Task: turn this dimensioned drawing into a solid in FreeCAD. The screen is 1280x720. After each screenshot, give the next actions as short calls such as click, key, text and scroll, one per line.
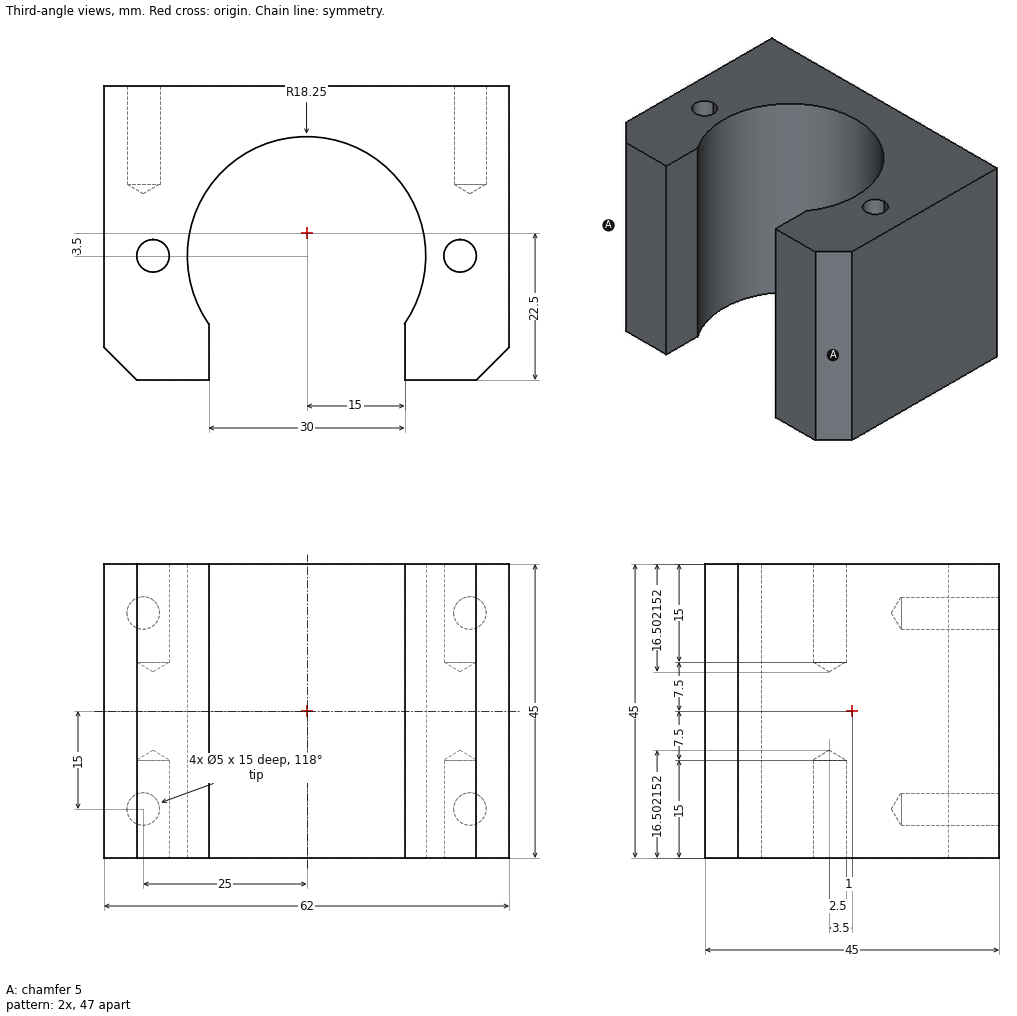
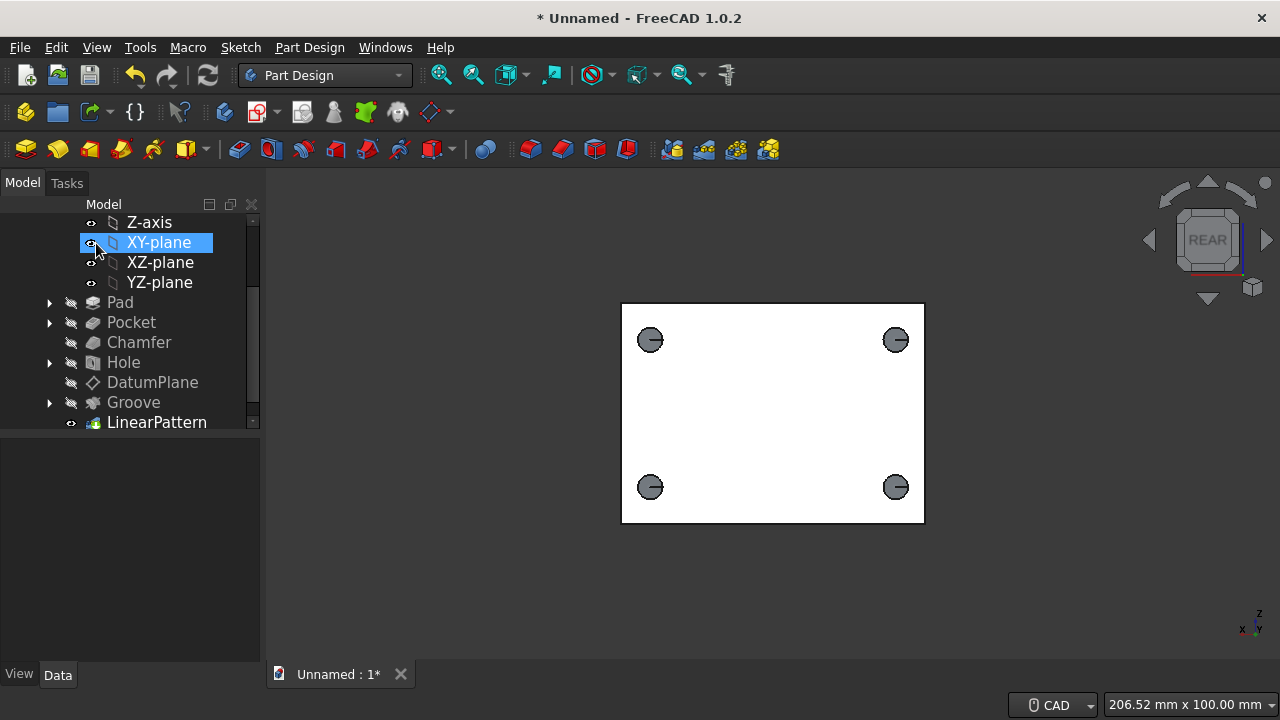
click(116, 403)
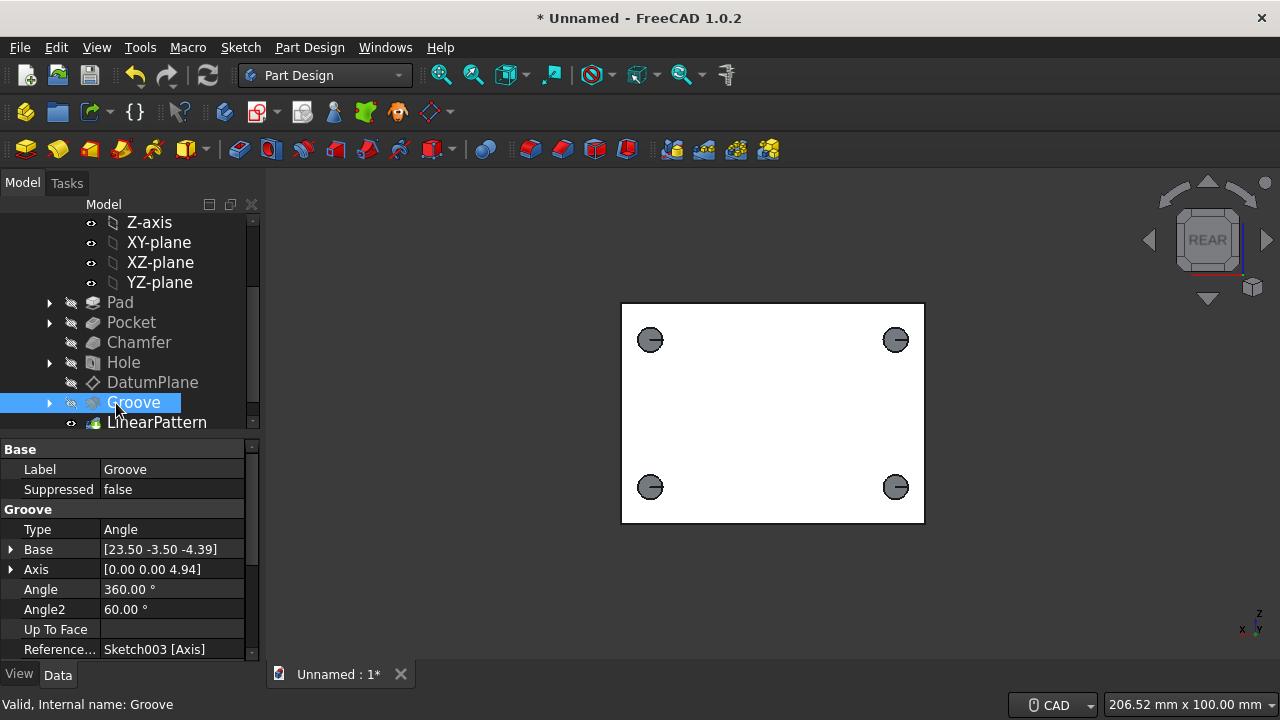
click(672, 150)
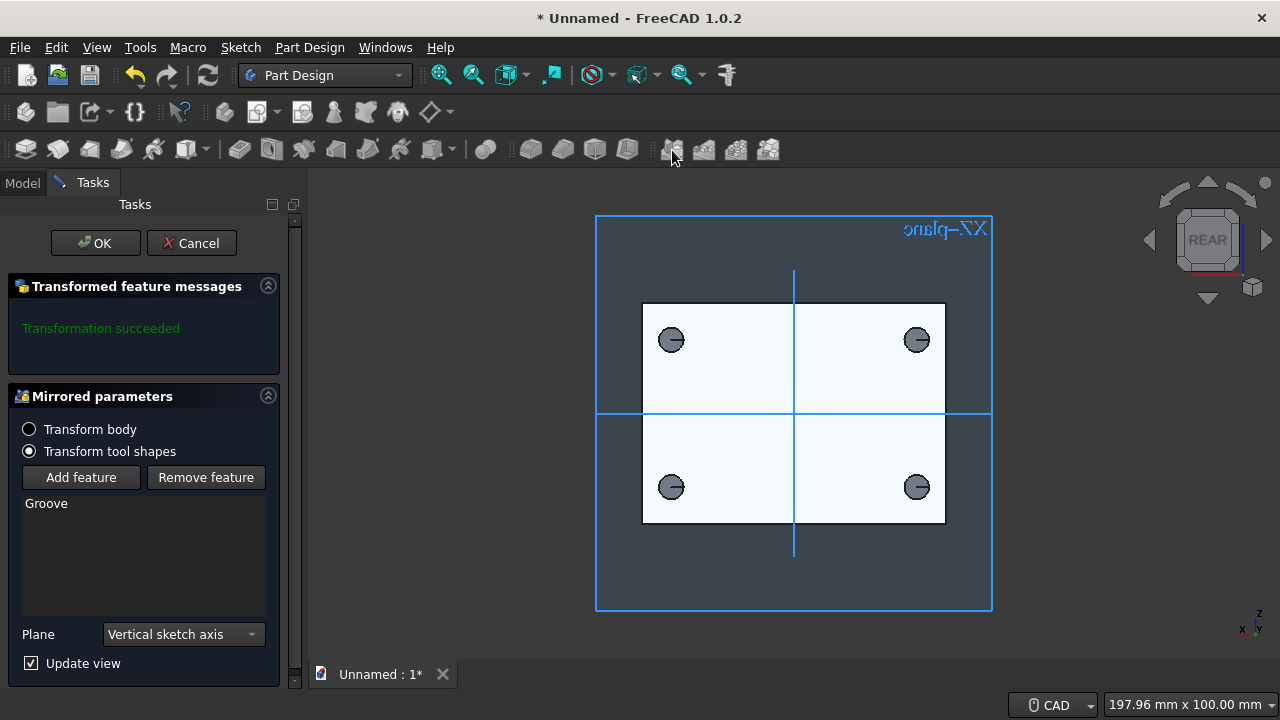
click(184, 634)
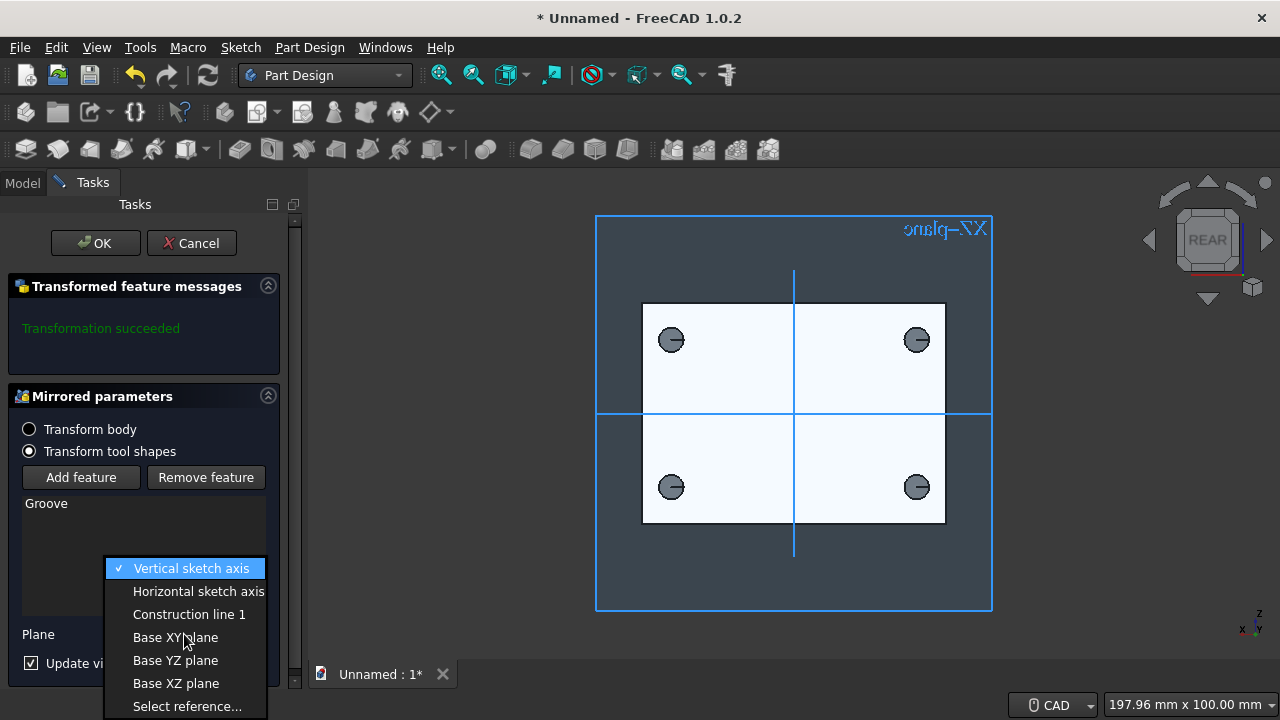
click(184, 638)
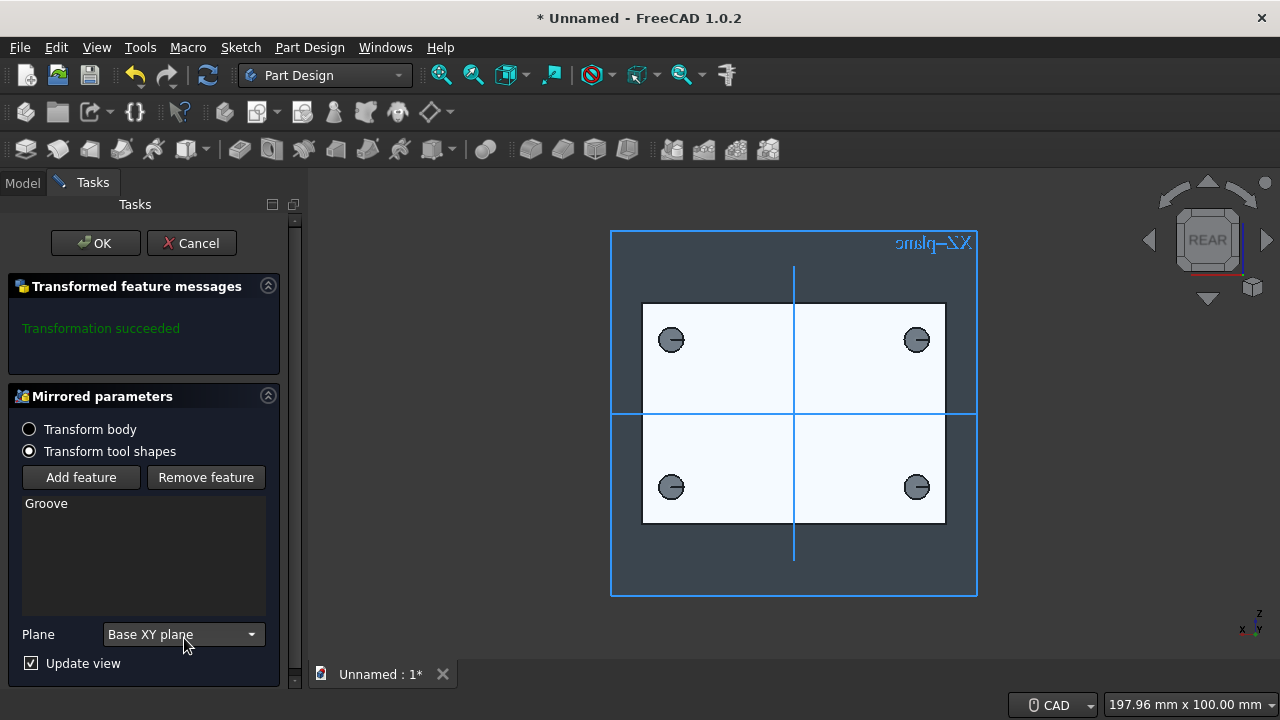
click(96, 243)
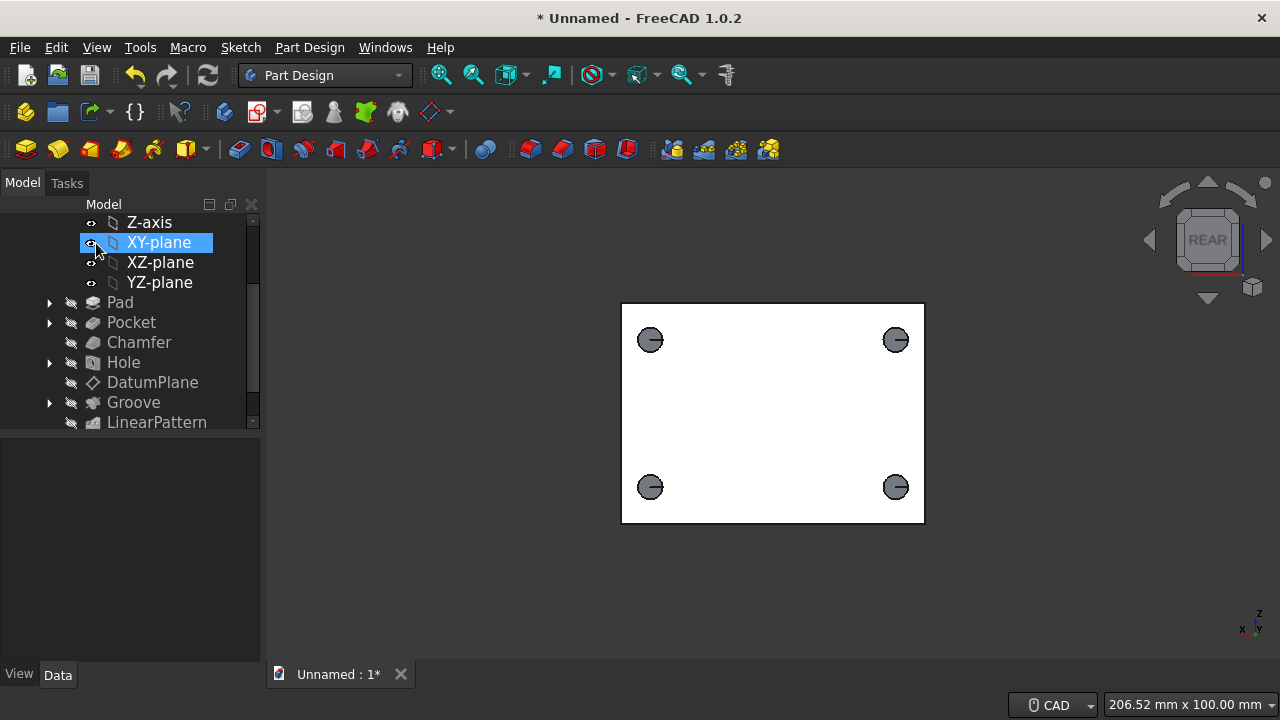
scroll(160, 318, down, 3)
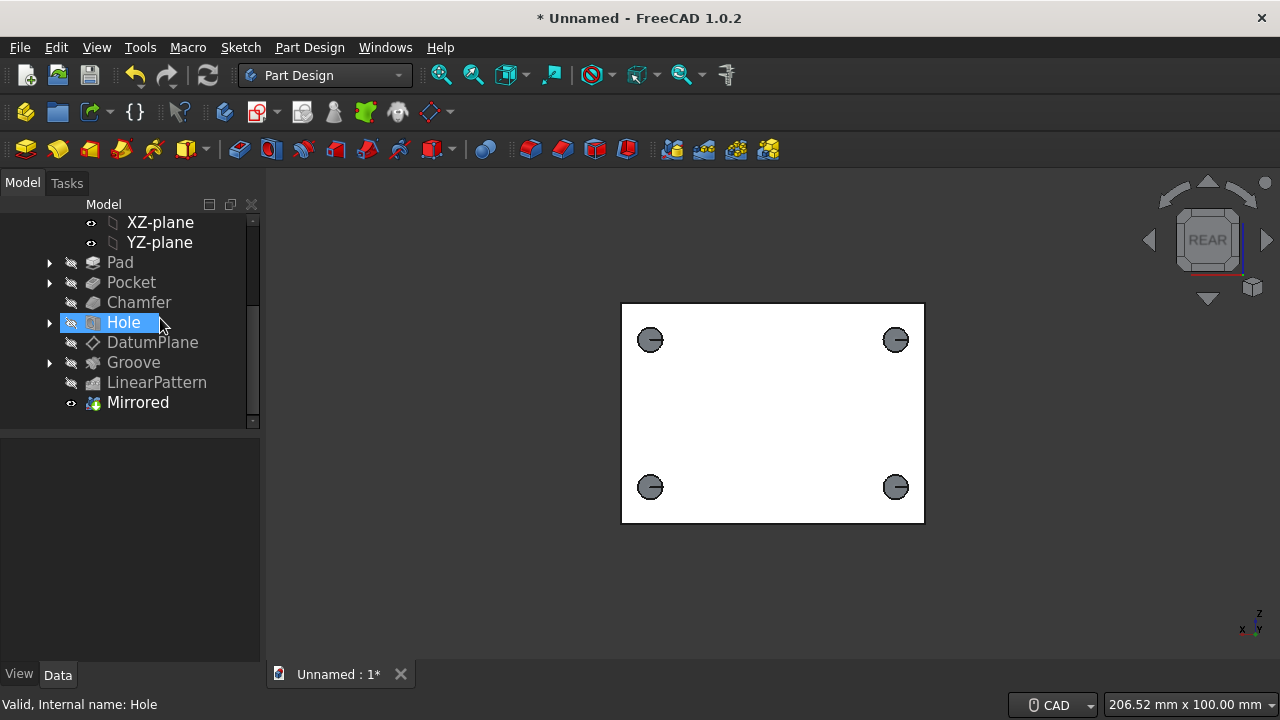
scroll(160, 318, up, 15)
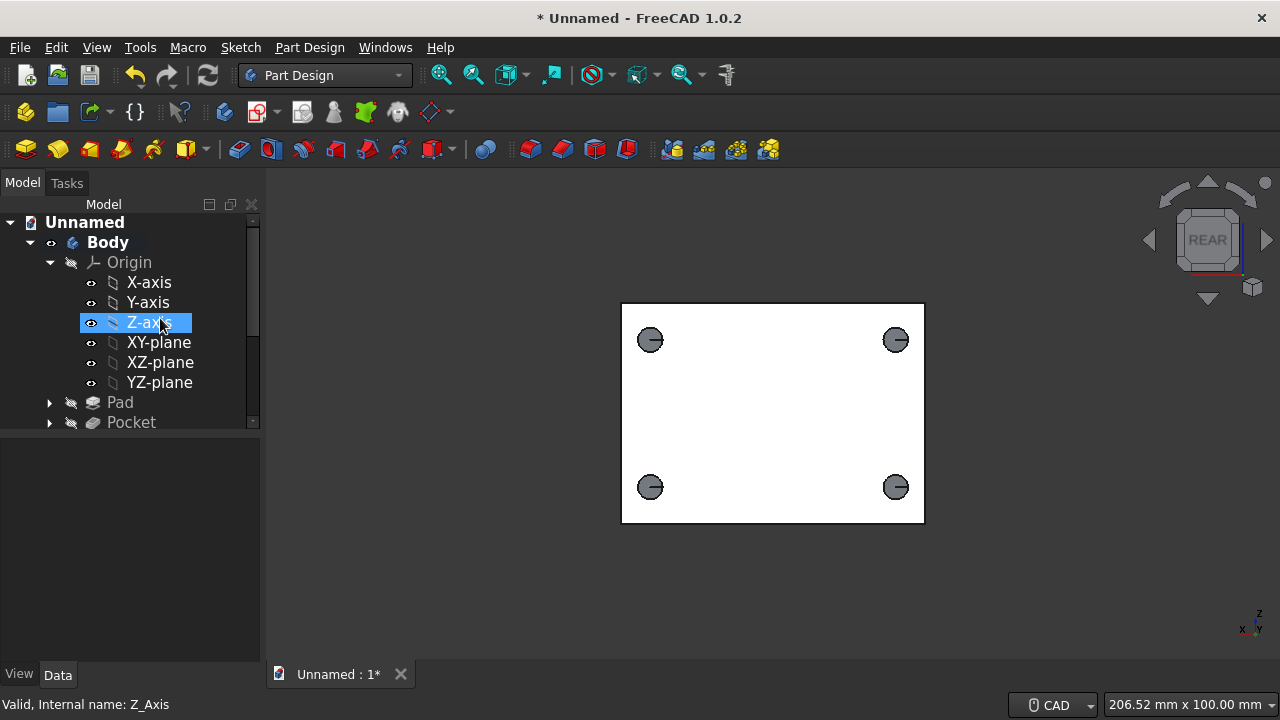
click(136, 383)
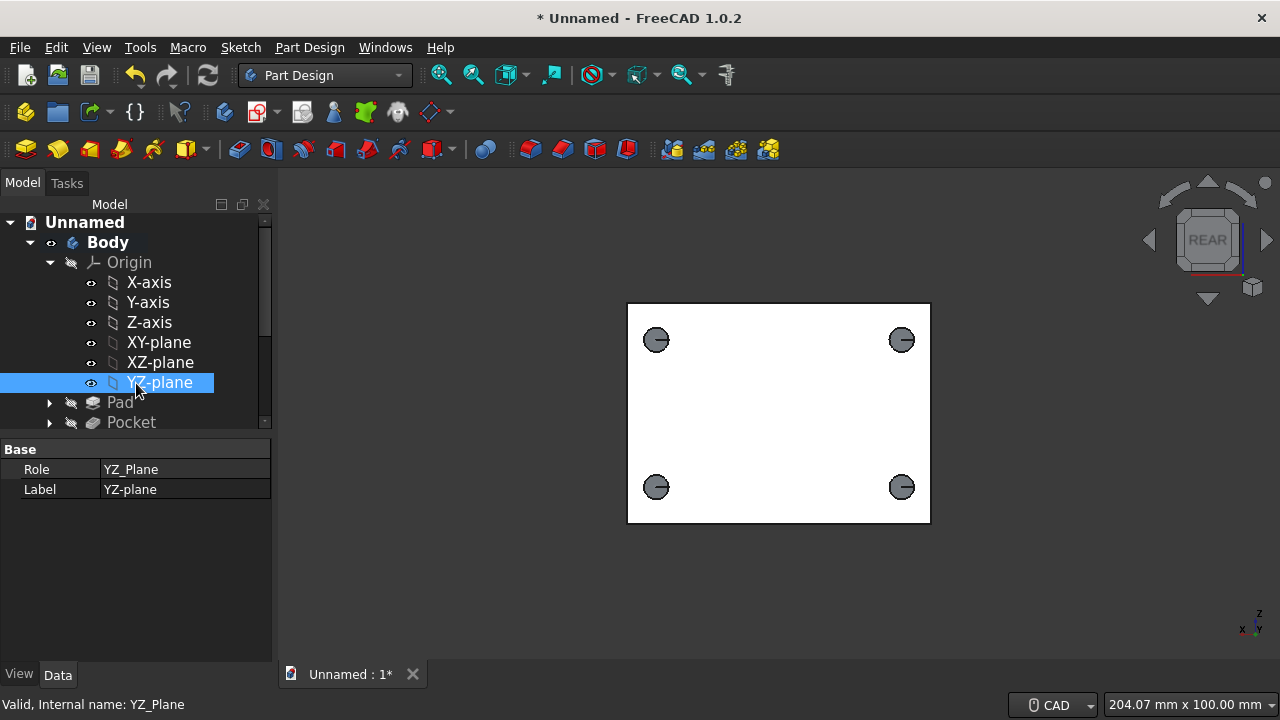
click(430, 112)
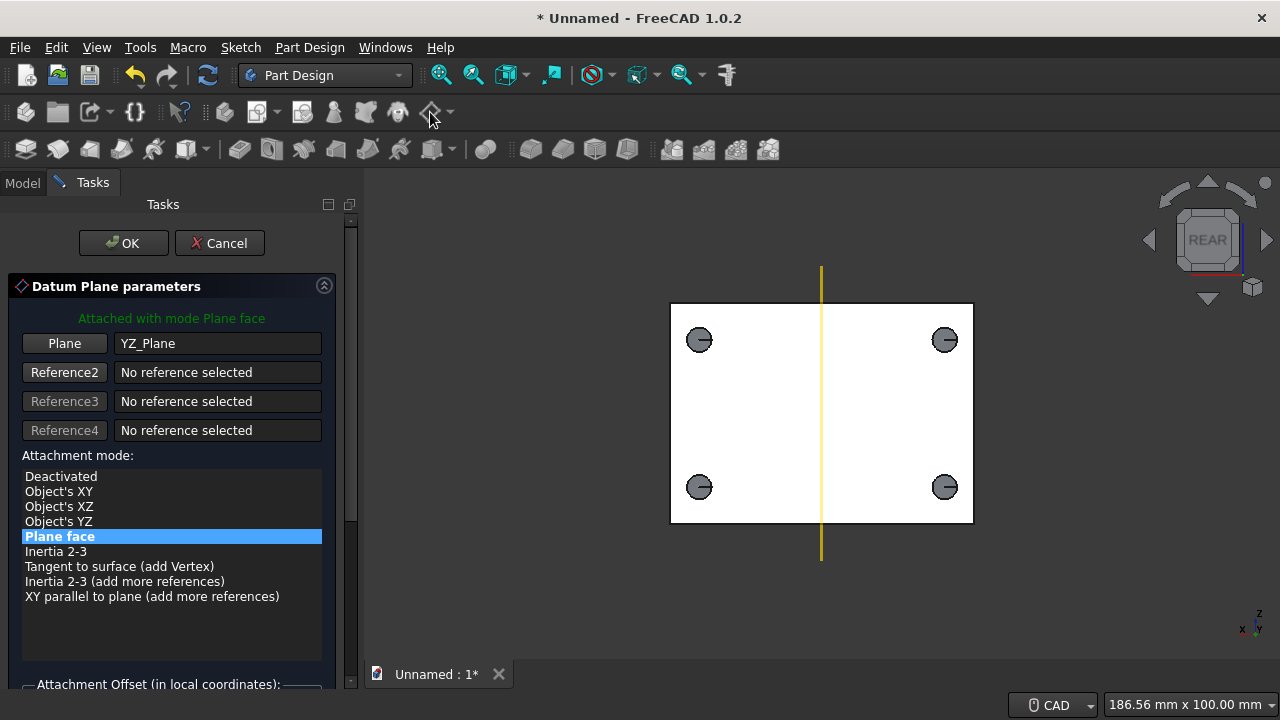
scroll(351, 451, down, 3)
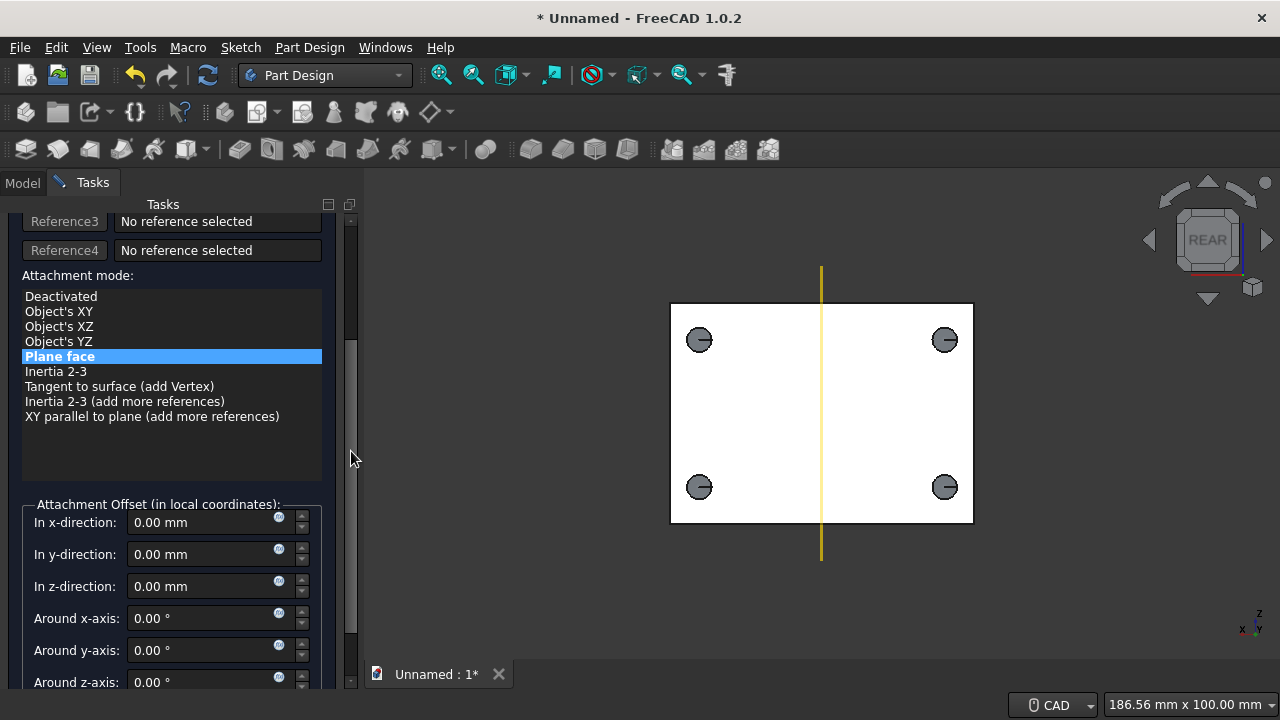
triple_click(210, 586)